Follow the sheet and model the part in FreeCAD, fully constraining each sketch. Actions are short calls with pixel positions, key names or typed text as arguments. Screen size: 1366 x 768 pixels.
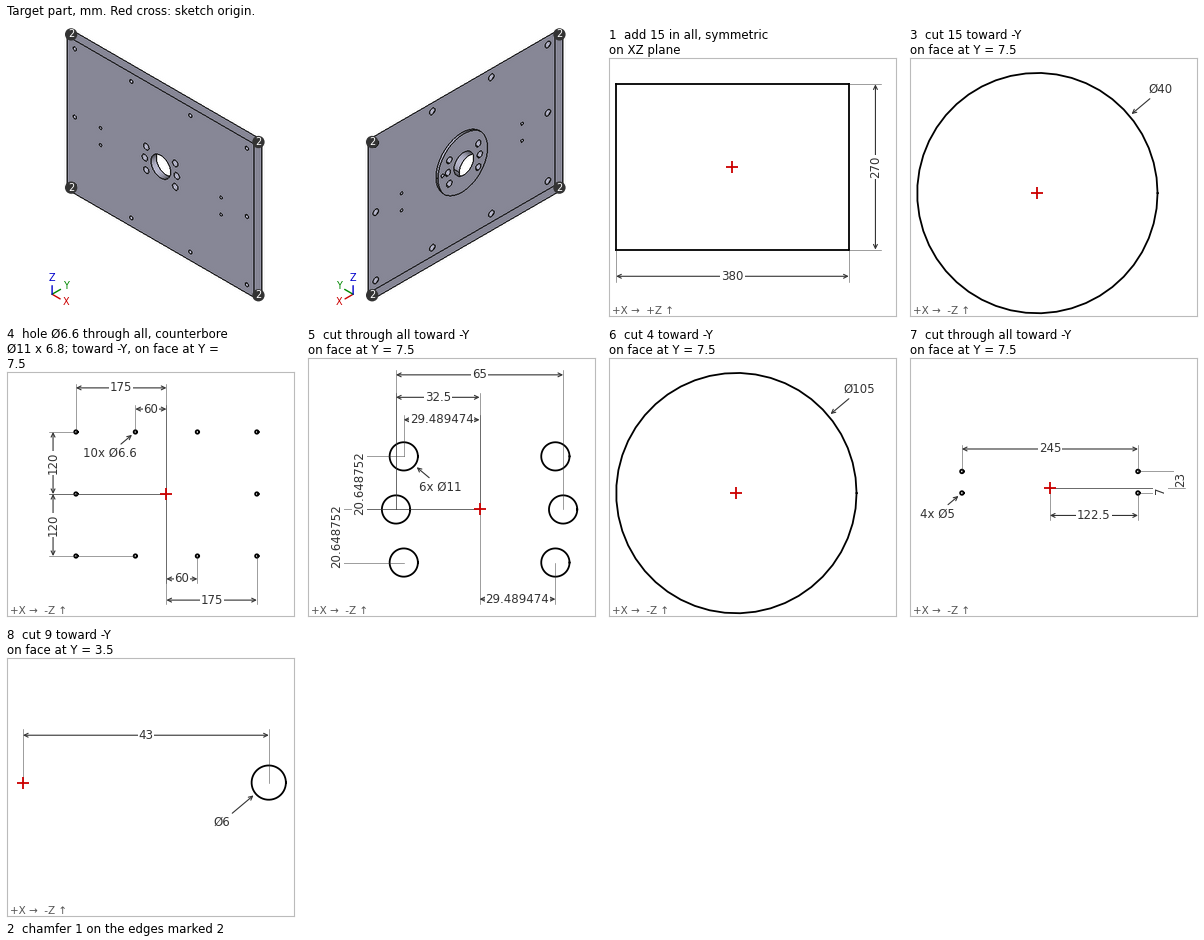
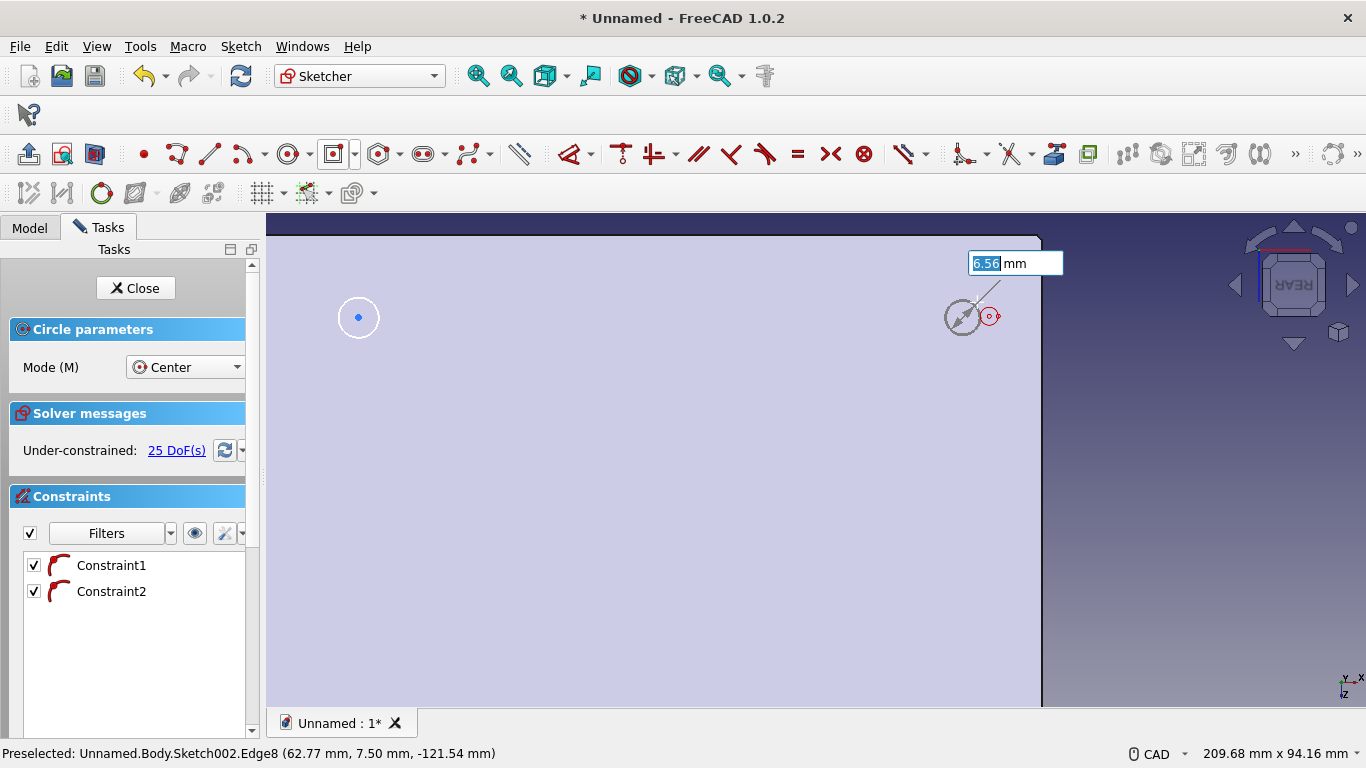
click(976, 302)
key(Escape)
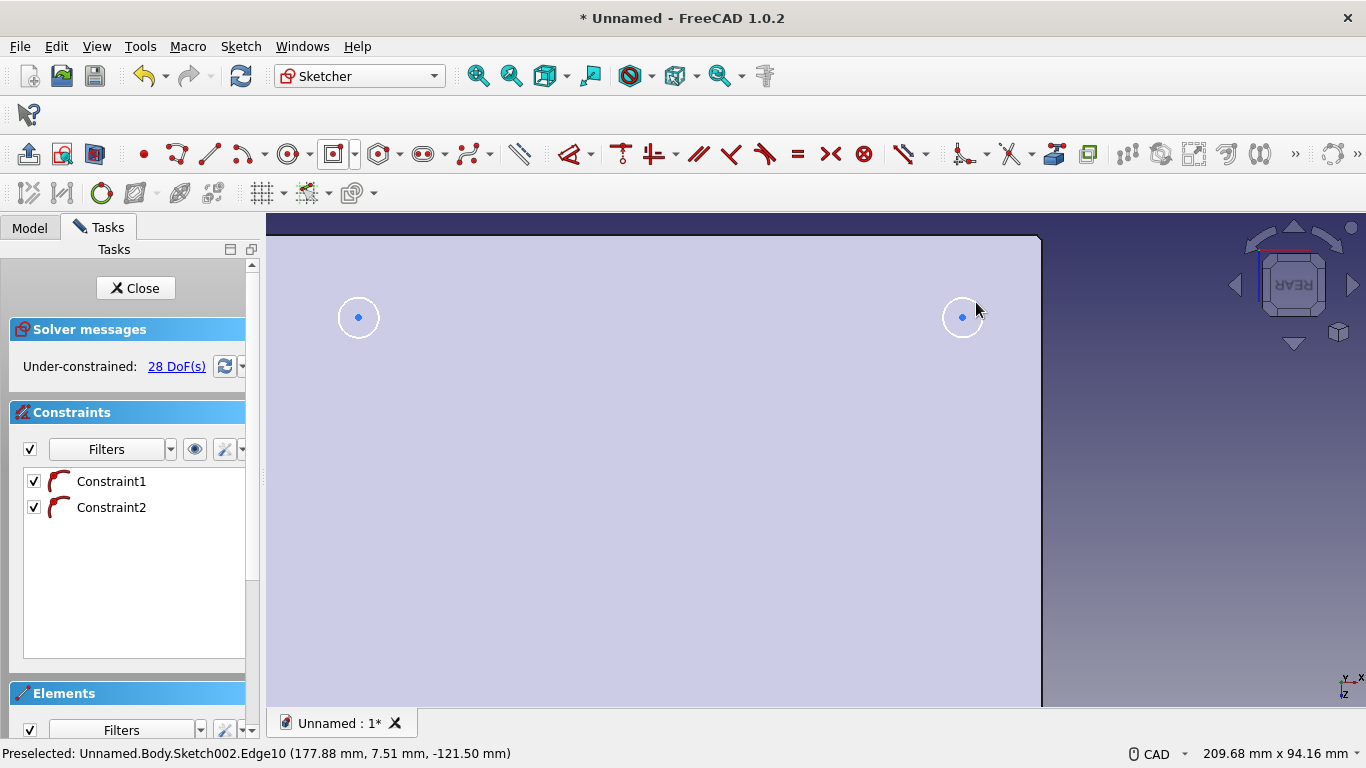
scroll(977, 302, down, 7)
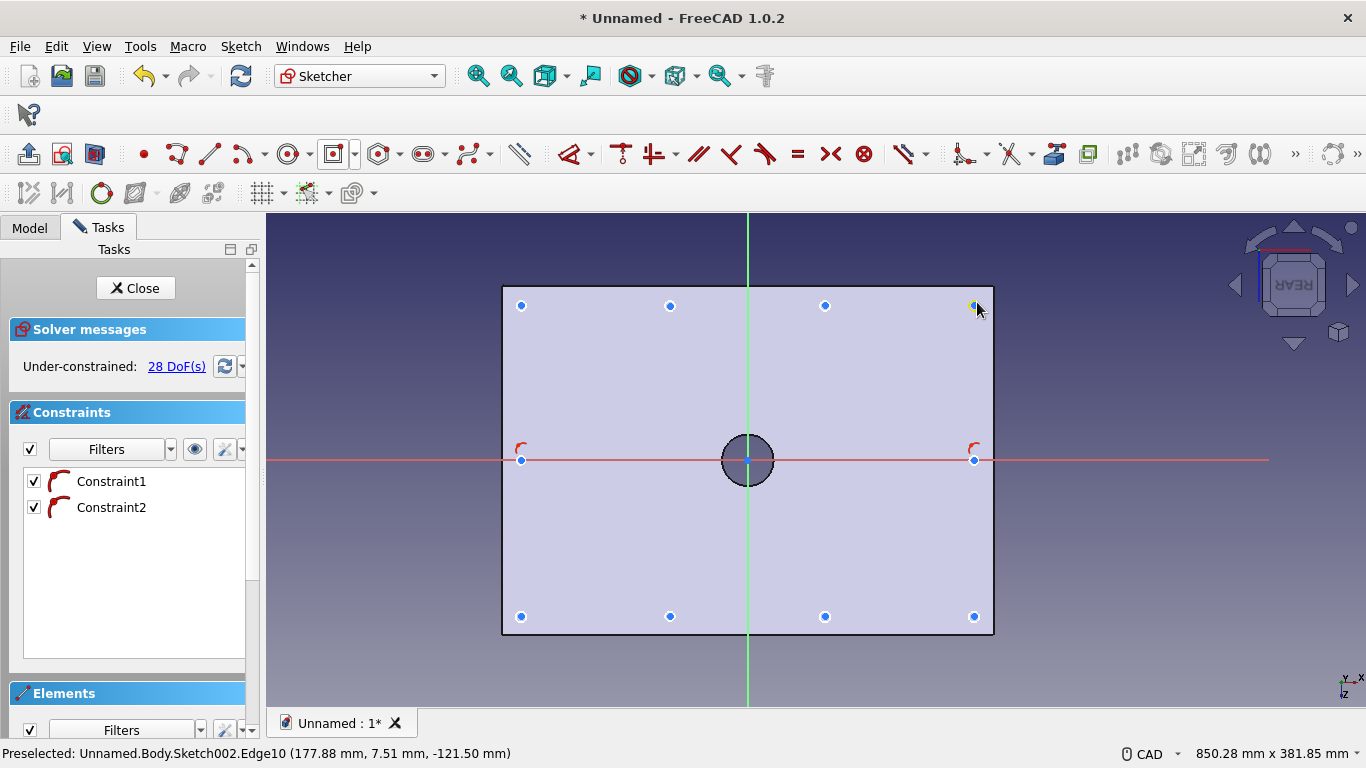
scroll(525, 302, up, 6)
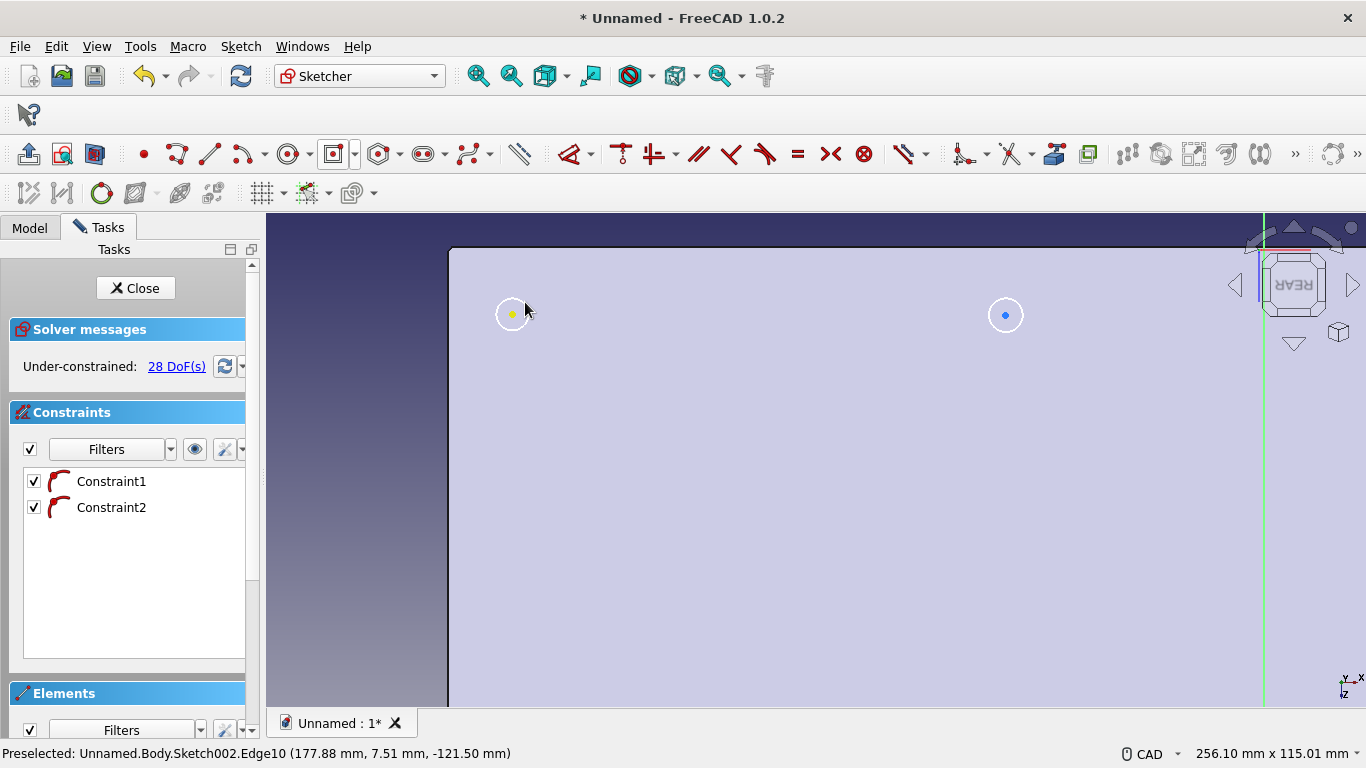
click(524, 303)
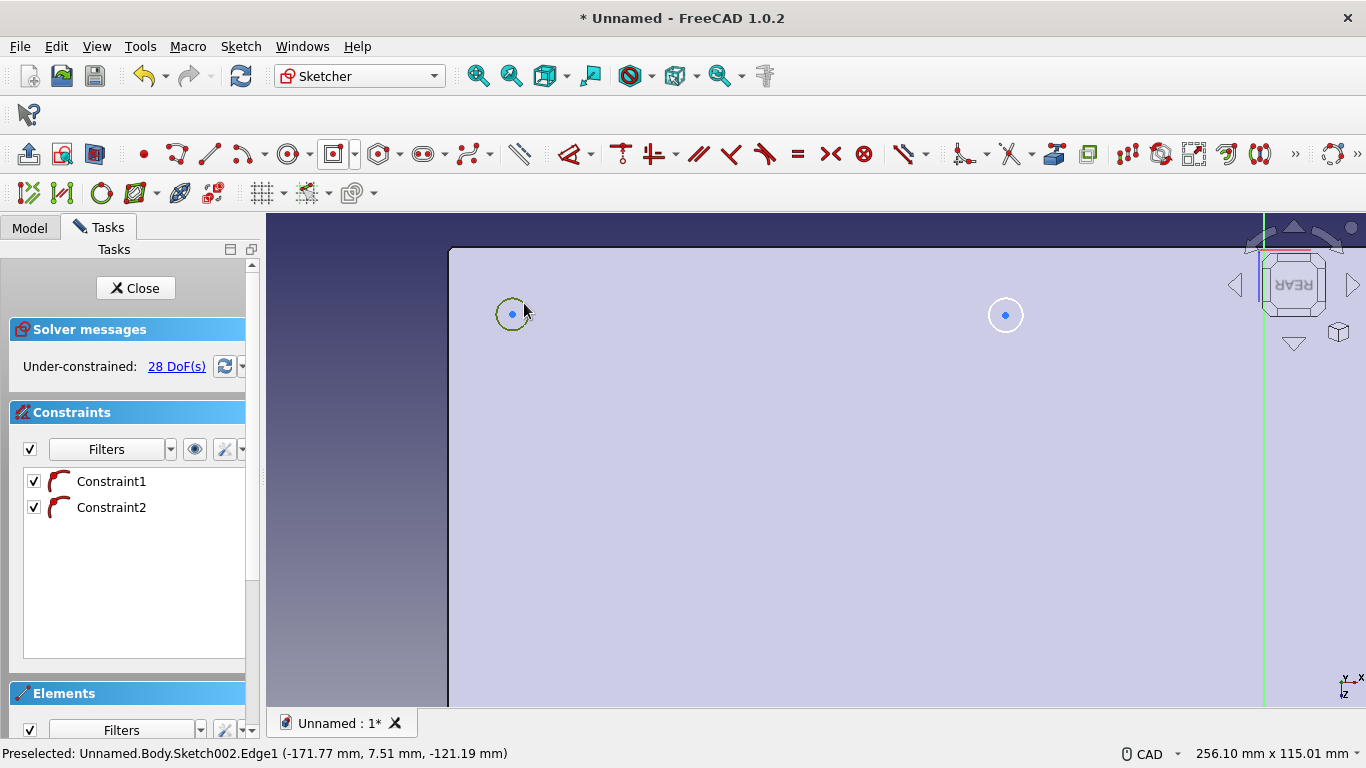
click(1018, 303)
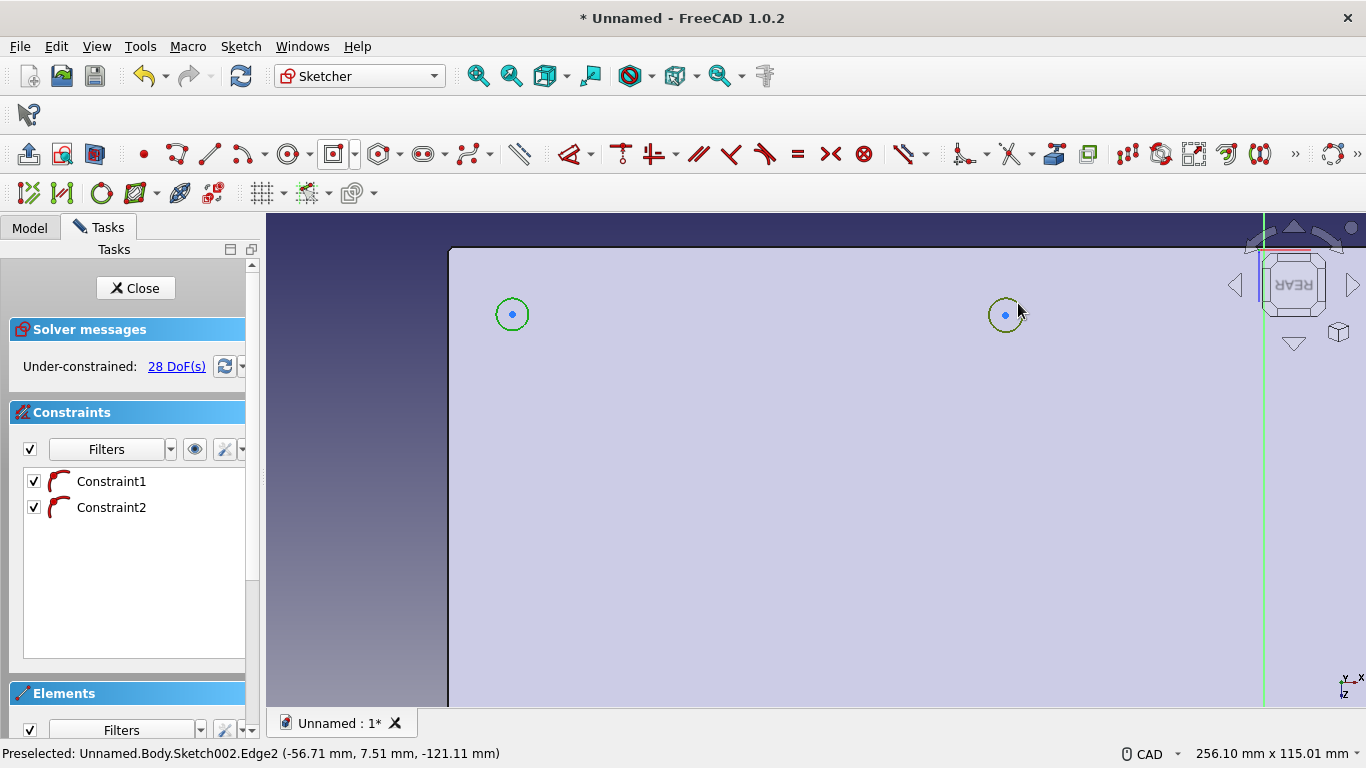
scroll(525, 302, down, 6)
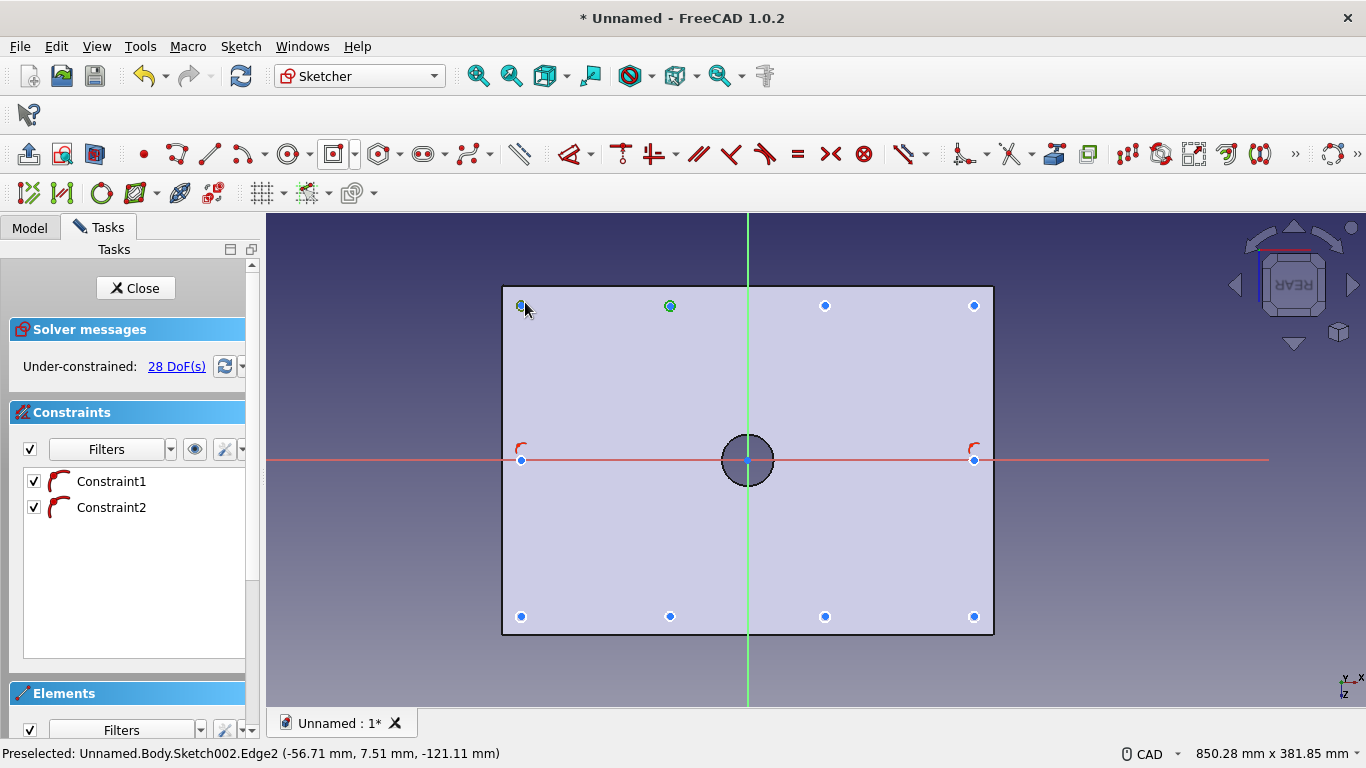
scroll(673, 613, up, 6)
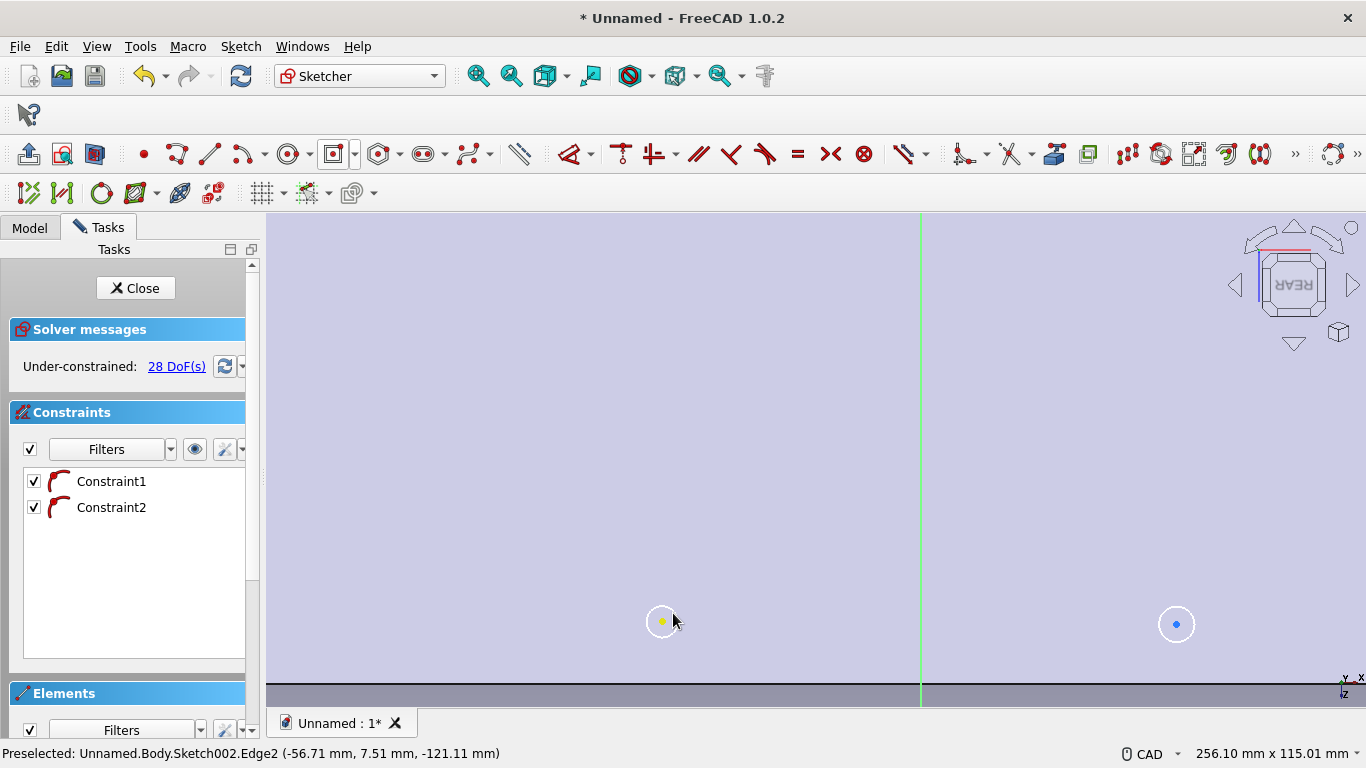
click(673, 611)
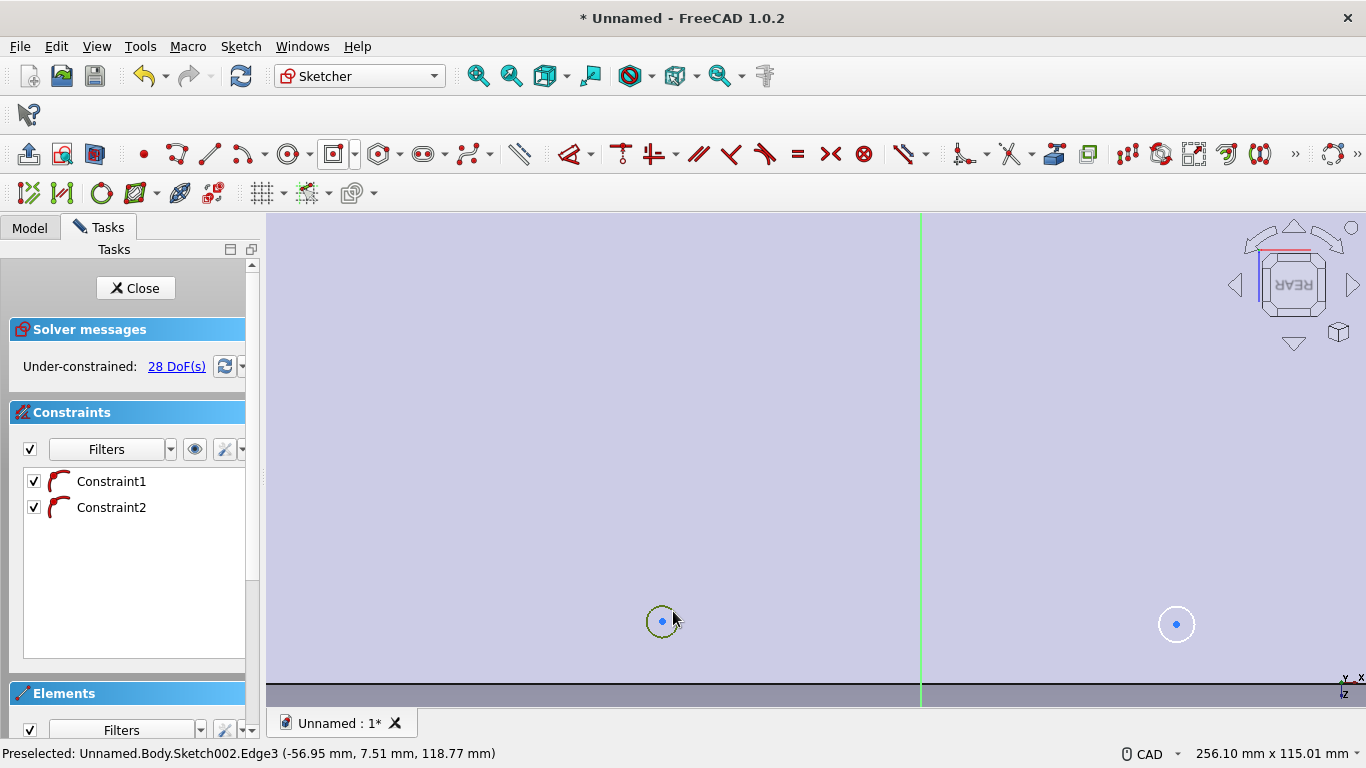
scroll(673, 613, down, 6)